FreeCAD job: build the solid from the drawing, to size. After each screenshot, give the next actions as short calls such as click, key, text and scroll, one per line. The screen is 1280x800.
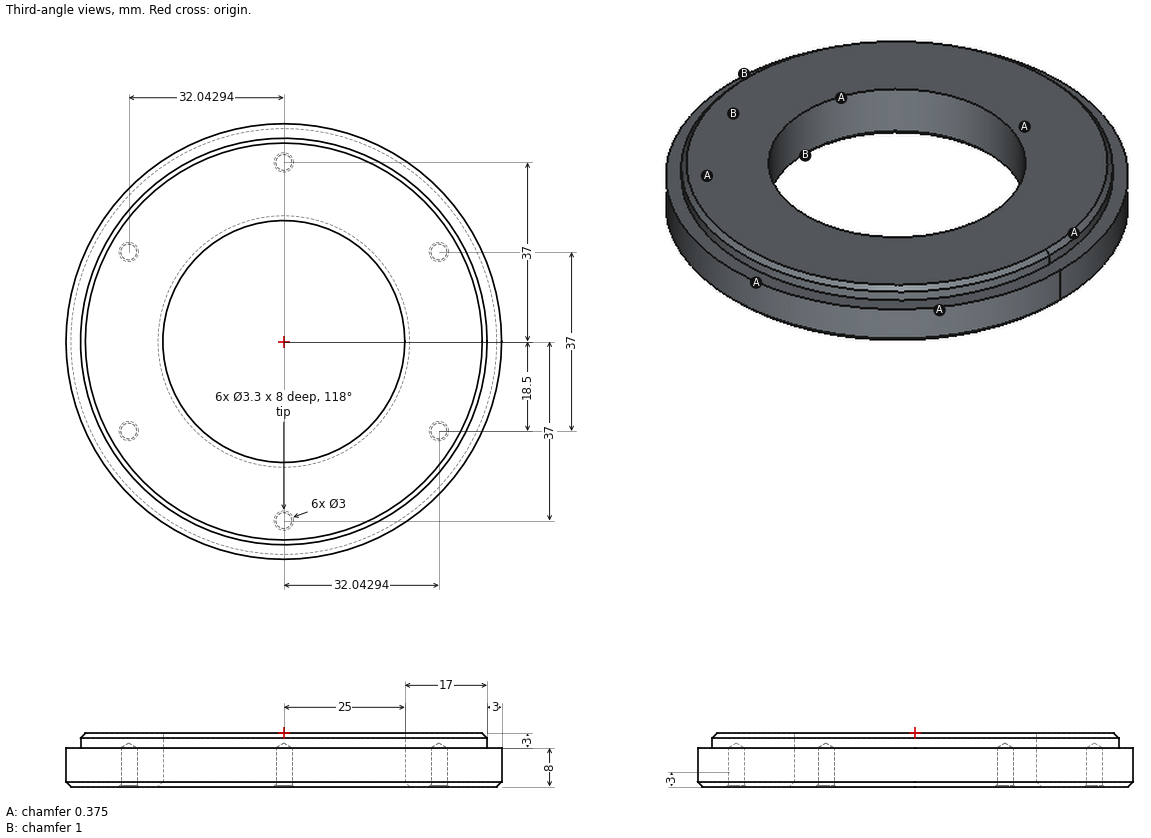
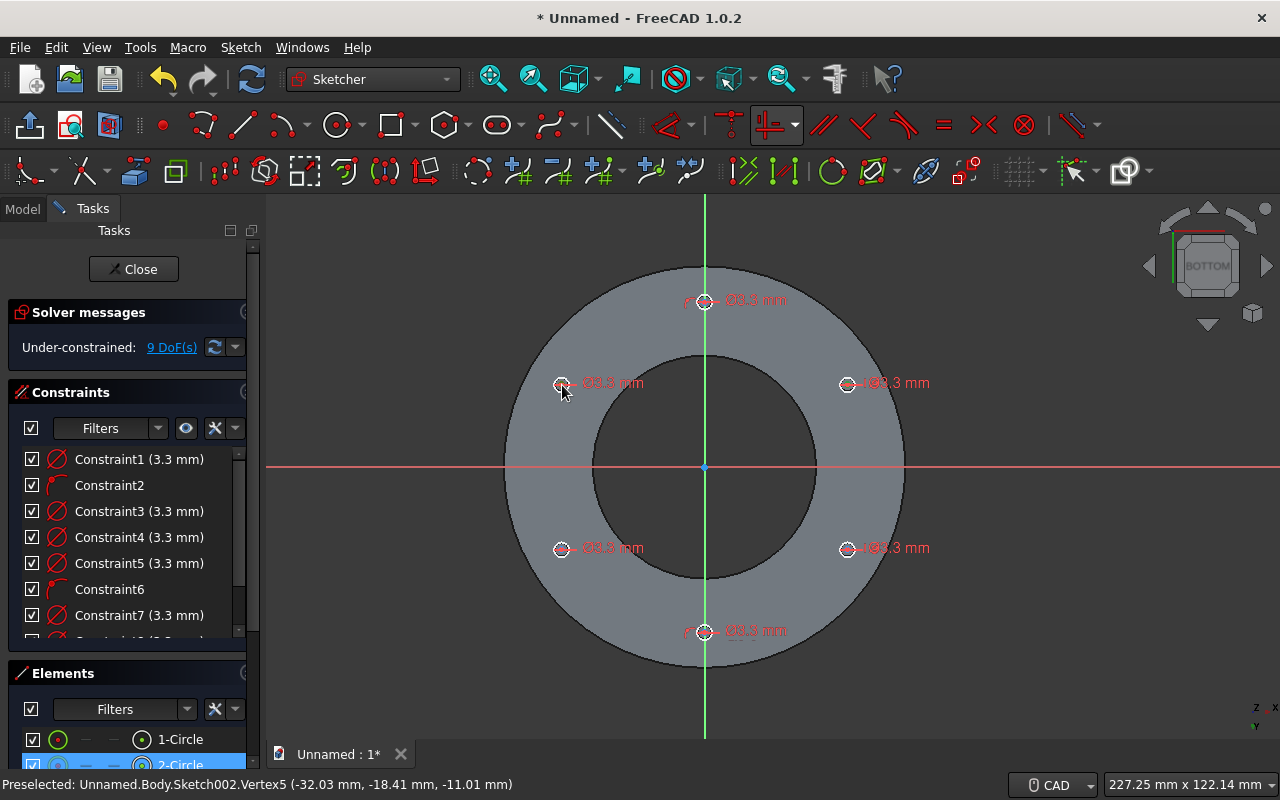
key(h)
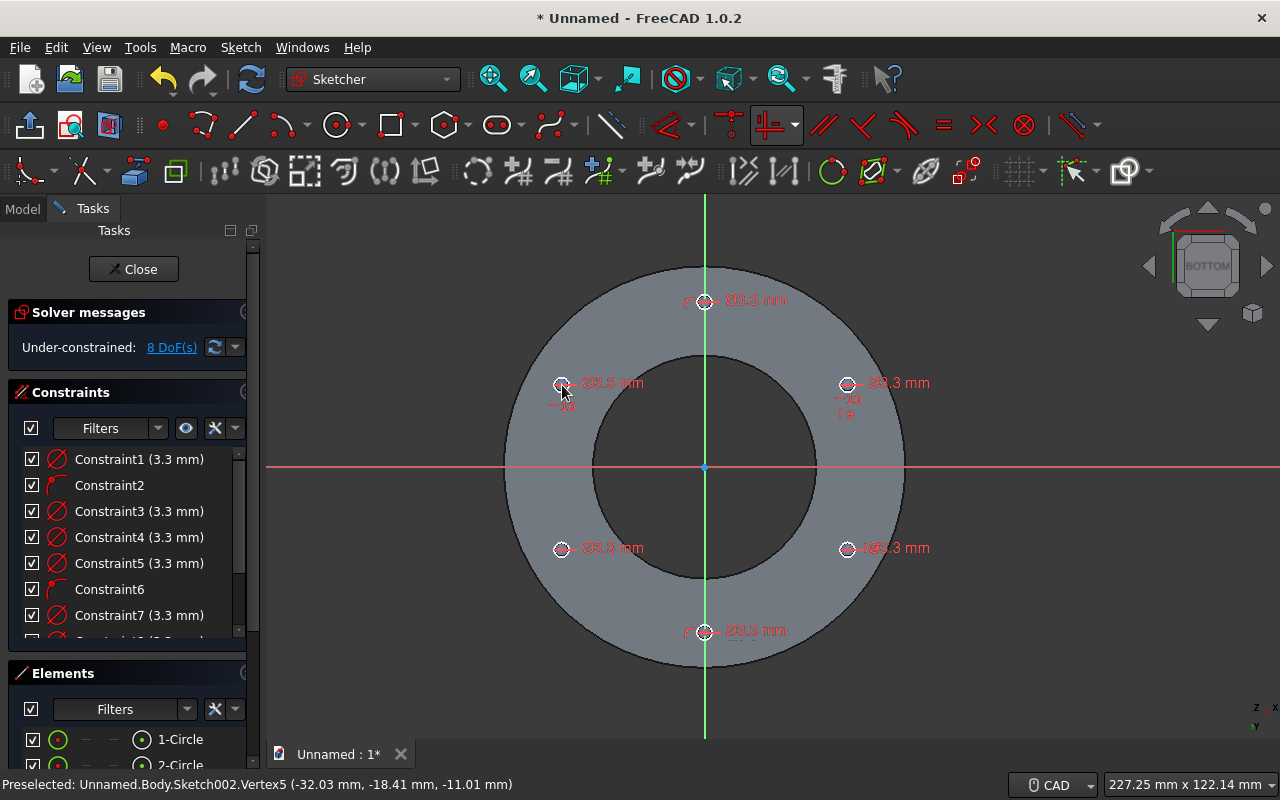
click(562, 385)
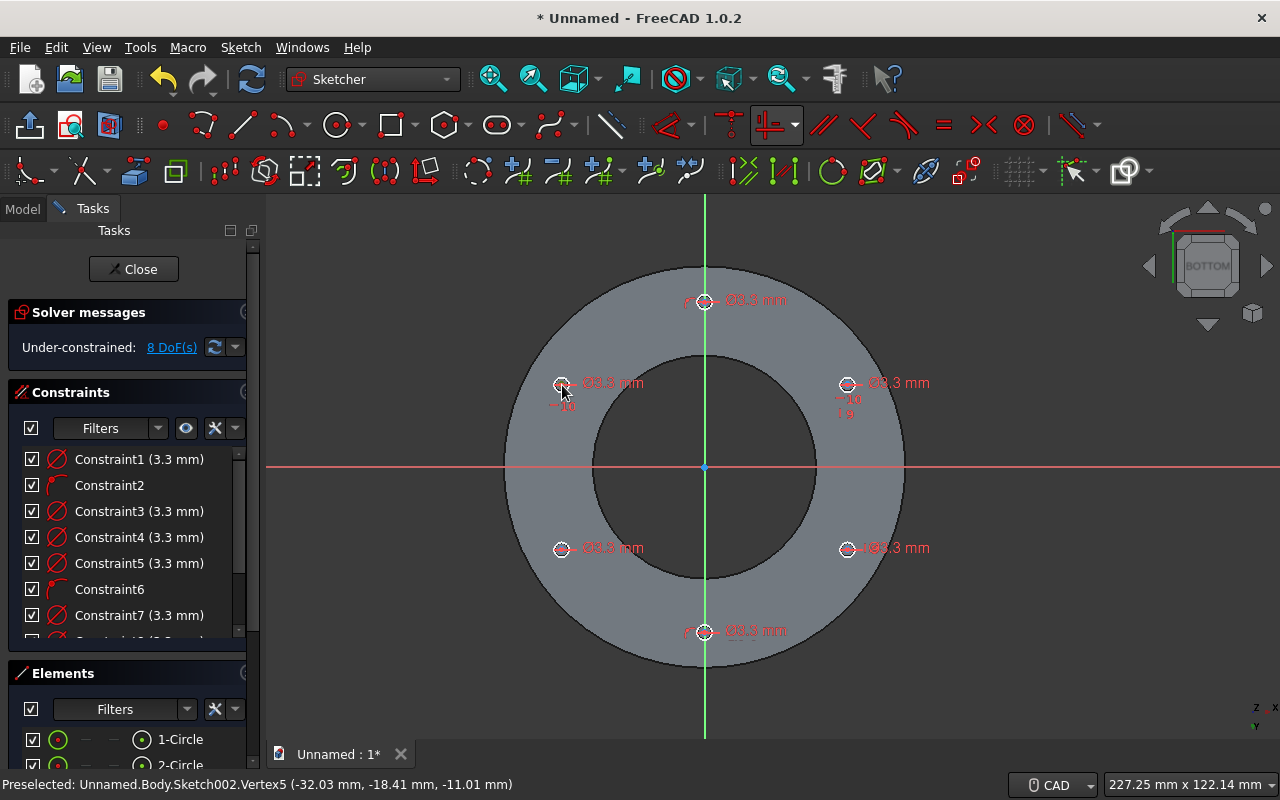
click(562, 550)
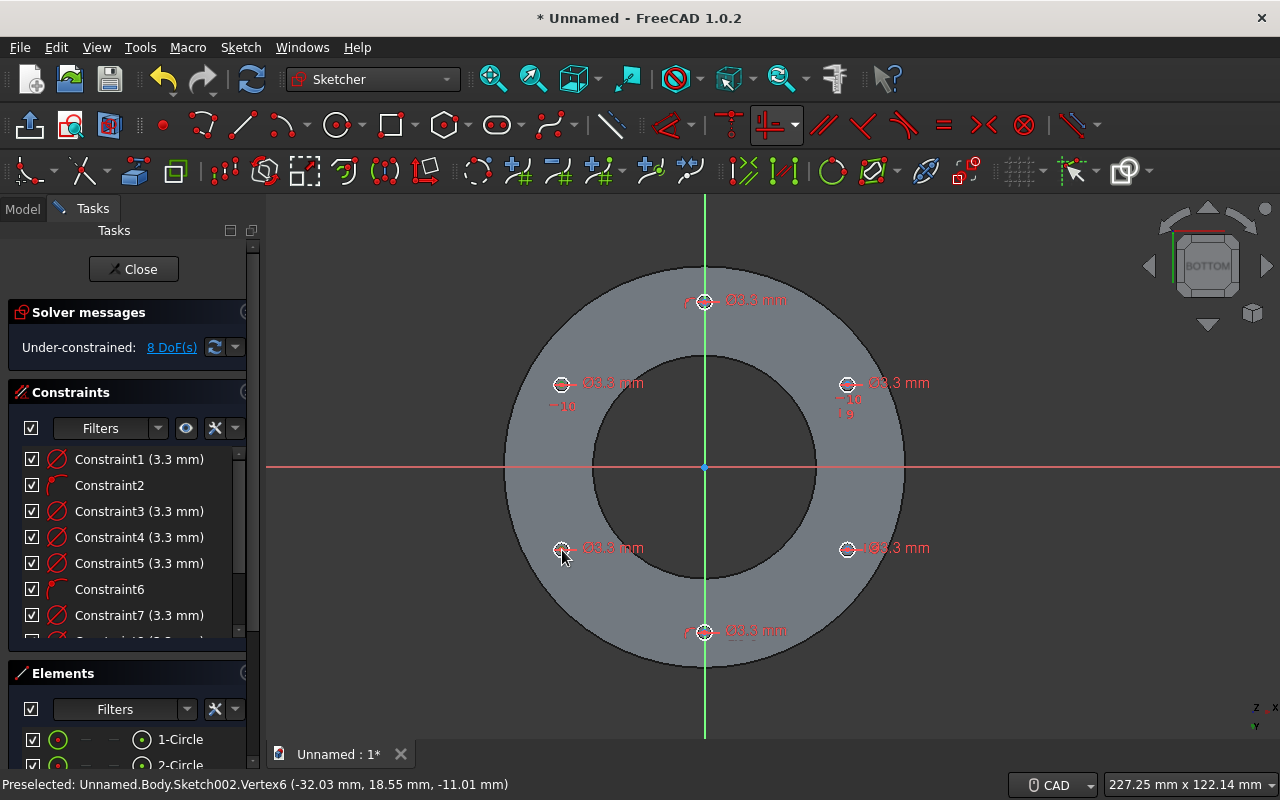
key(v)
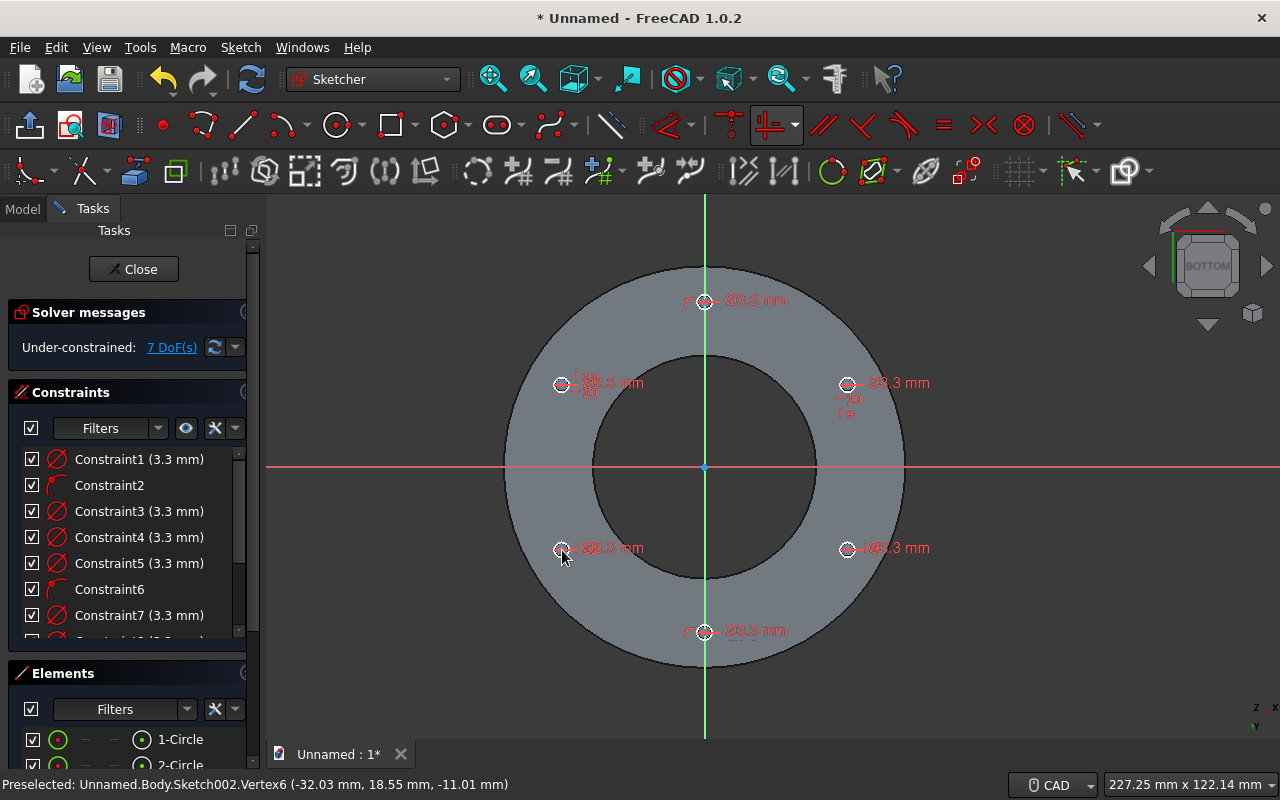
click(847, 550)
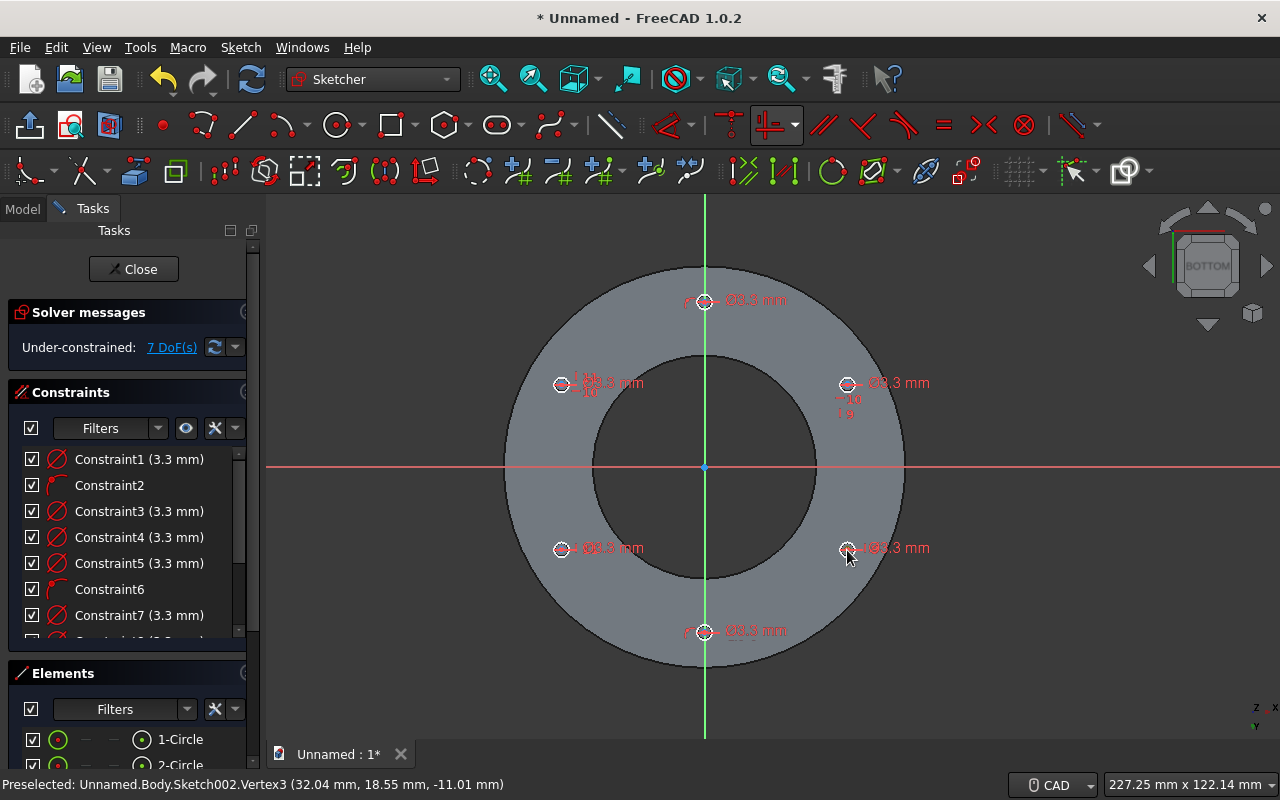
click(562, 550)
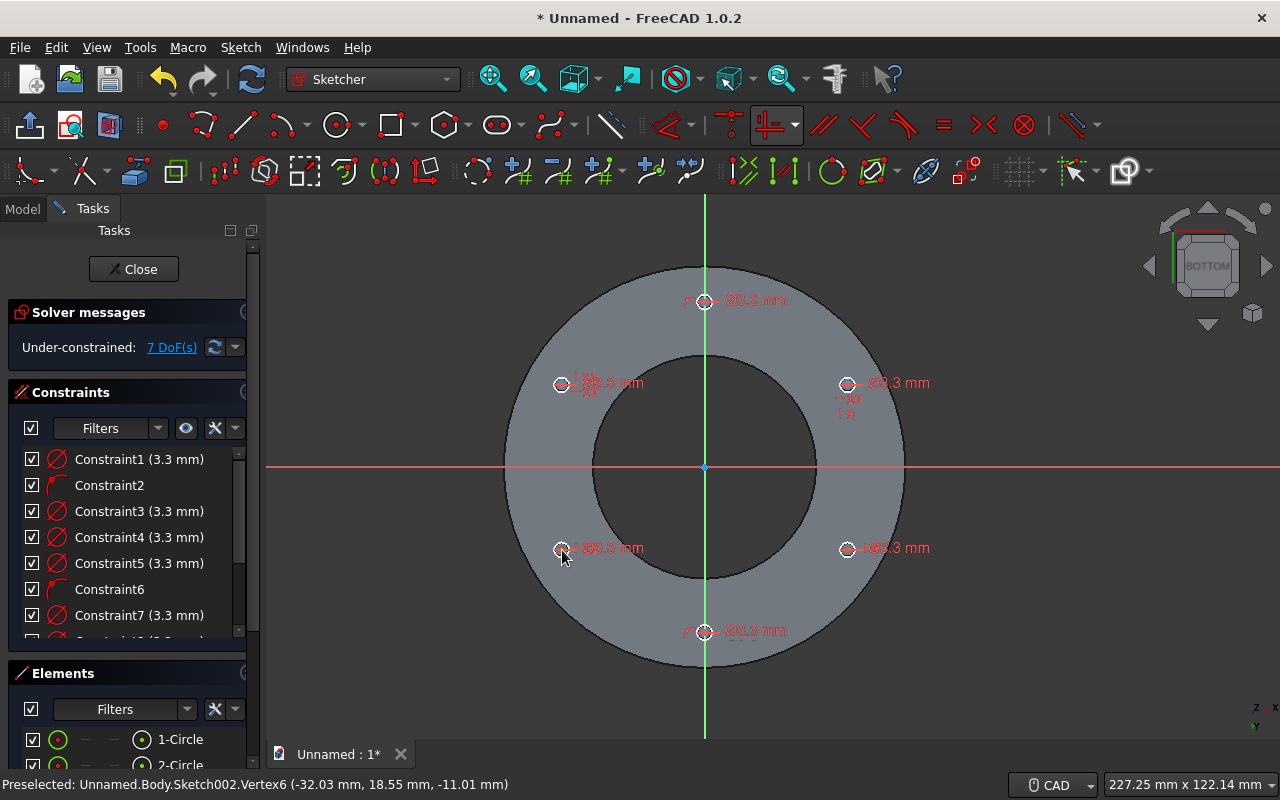
key(h)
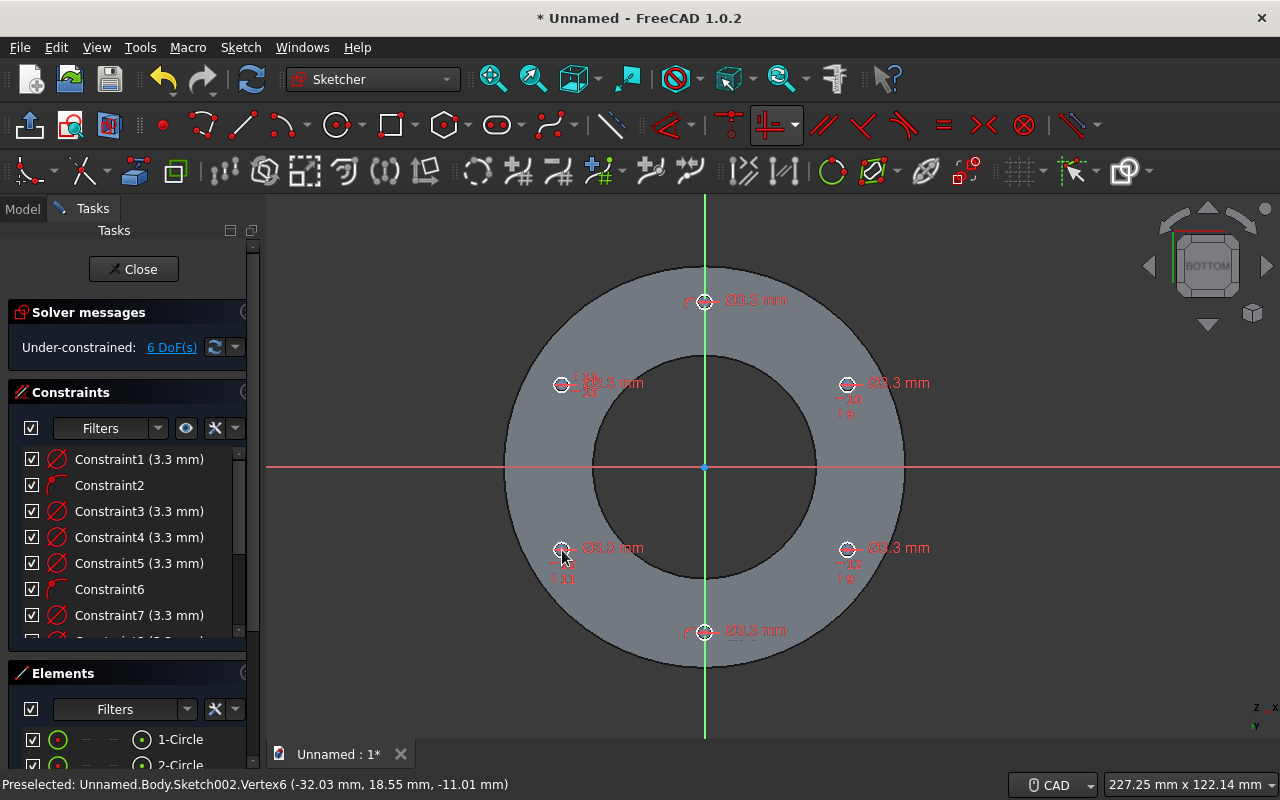
click(666, 126)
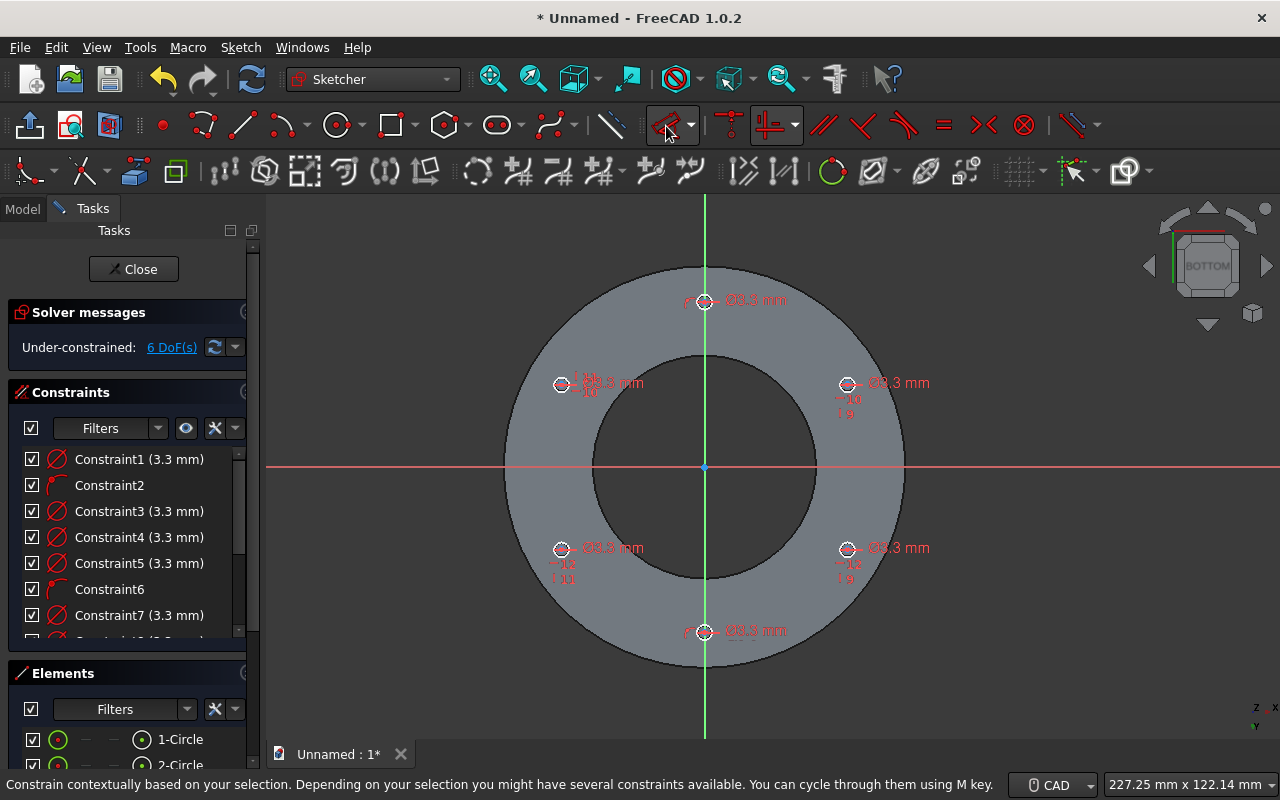
click(705, 302)
click(739, 385)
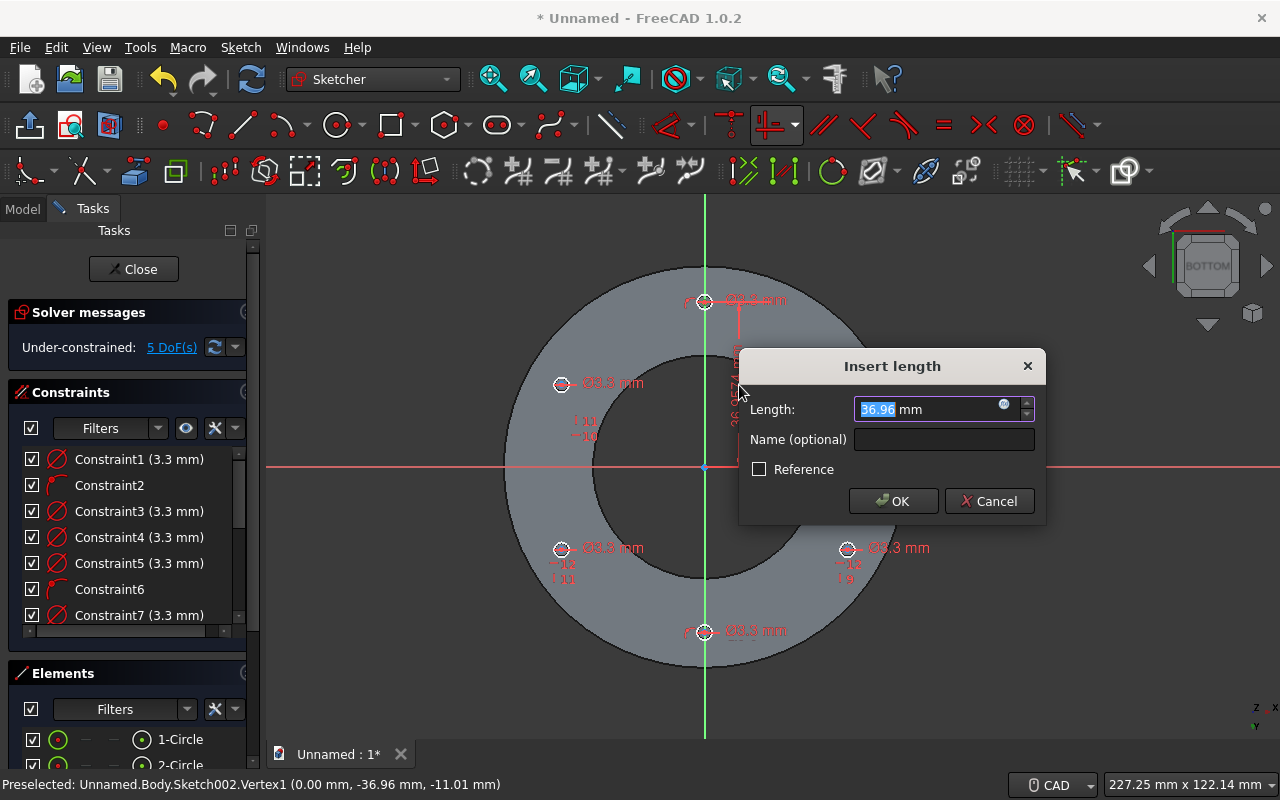
text(37)
key(Return)